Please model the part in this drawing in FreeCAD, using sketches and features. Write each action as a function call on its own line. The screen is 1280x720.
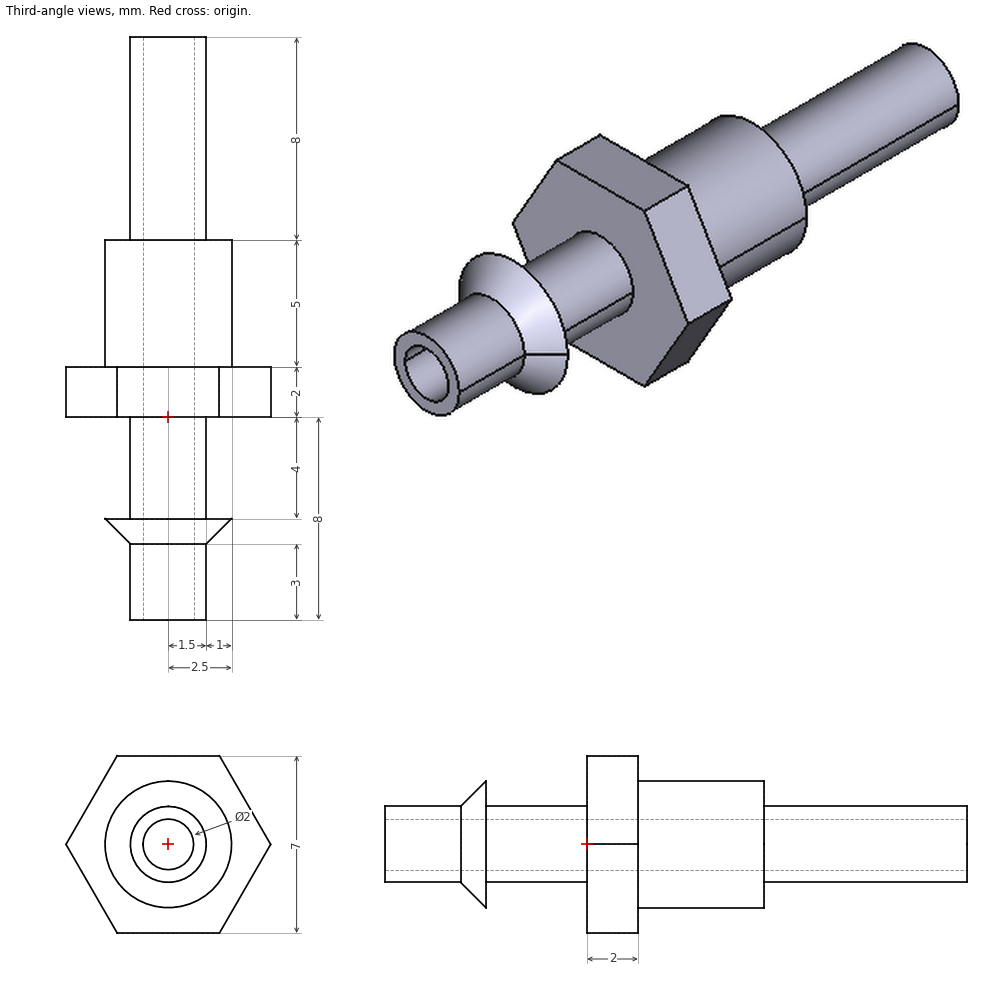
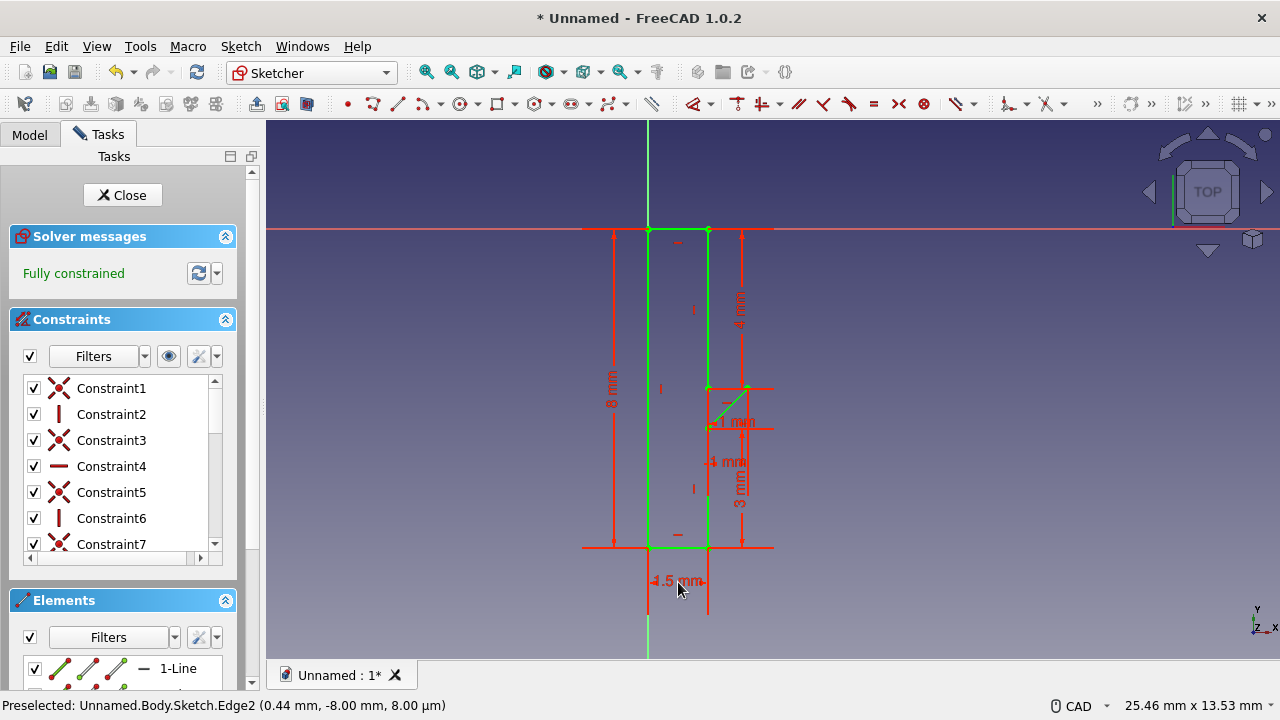
click(123, 195)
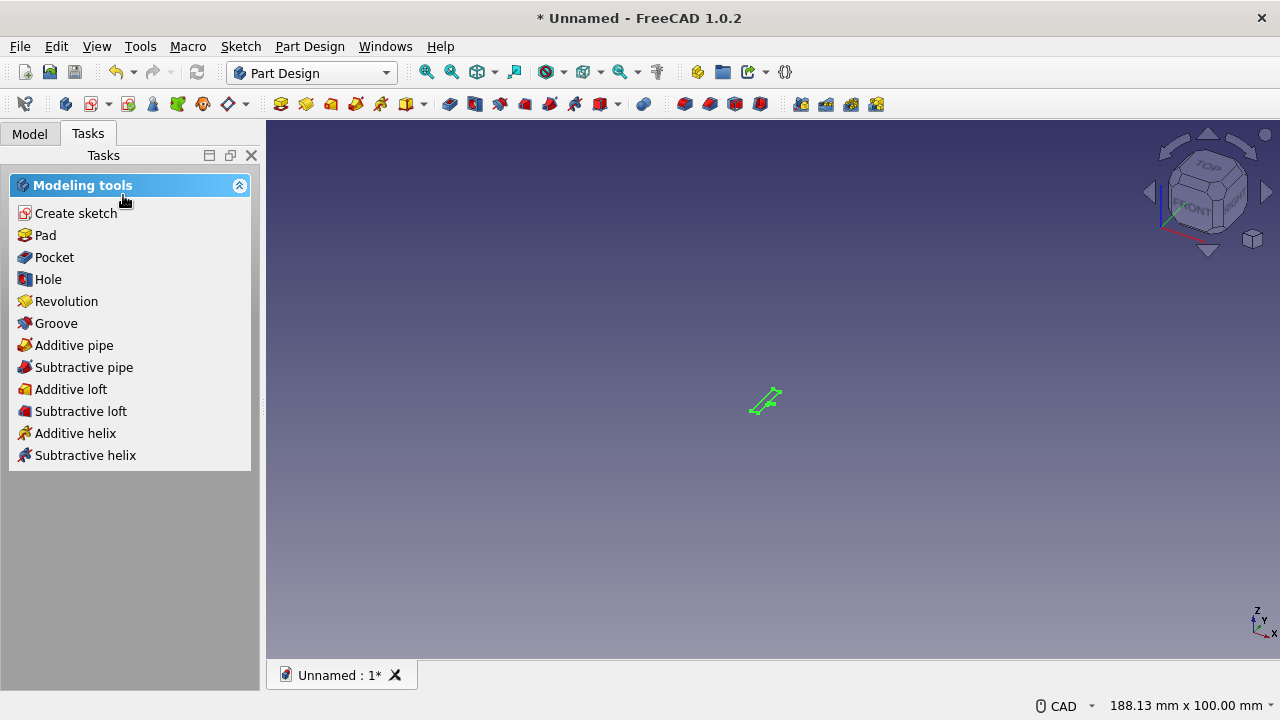
click(306, 104)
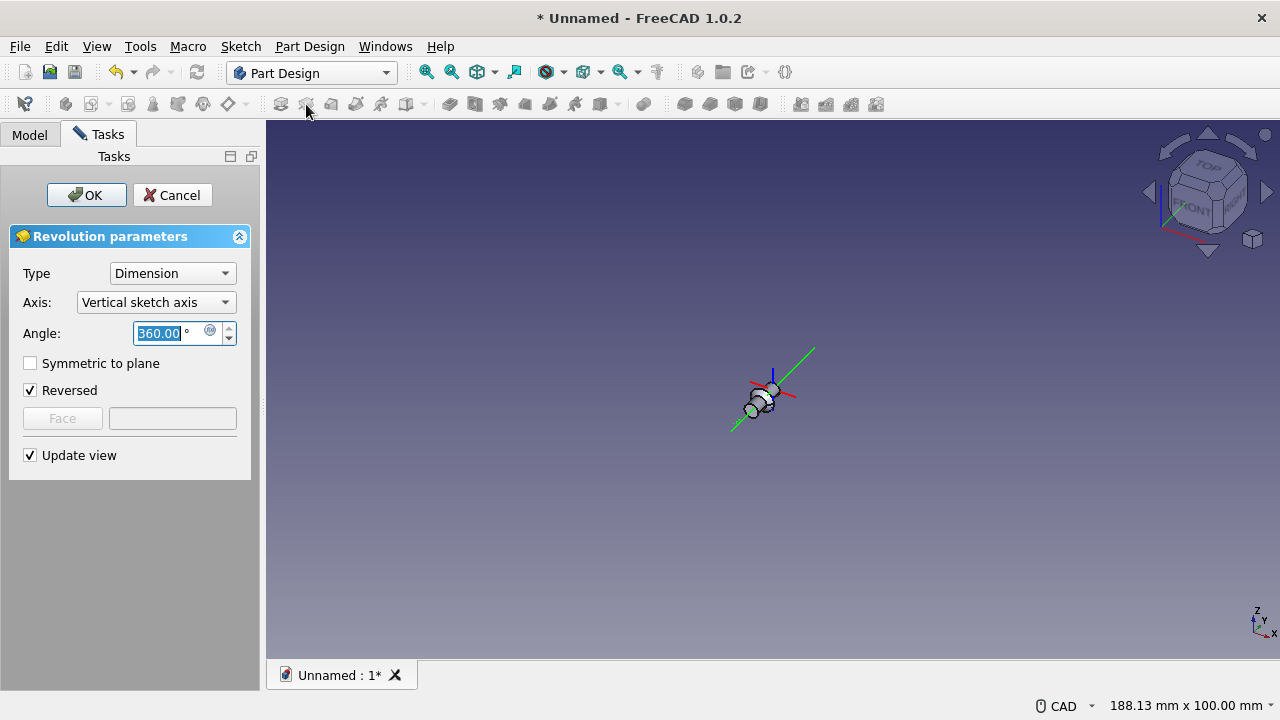
click(87, 195)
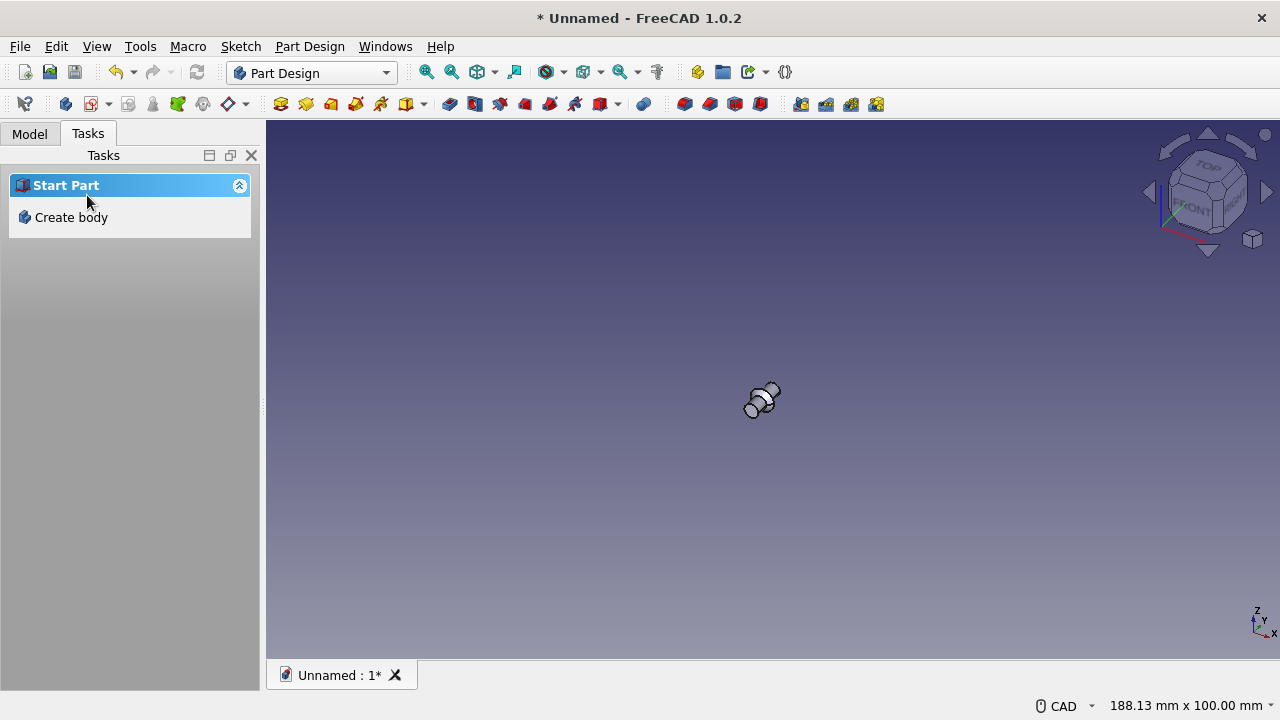
click(427, 72)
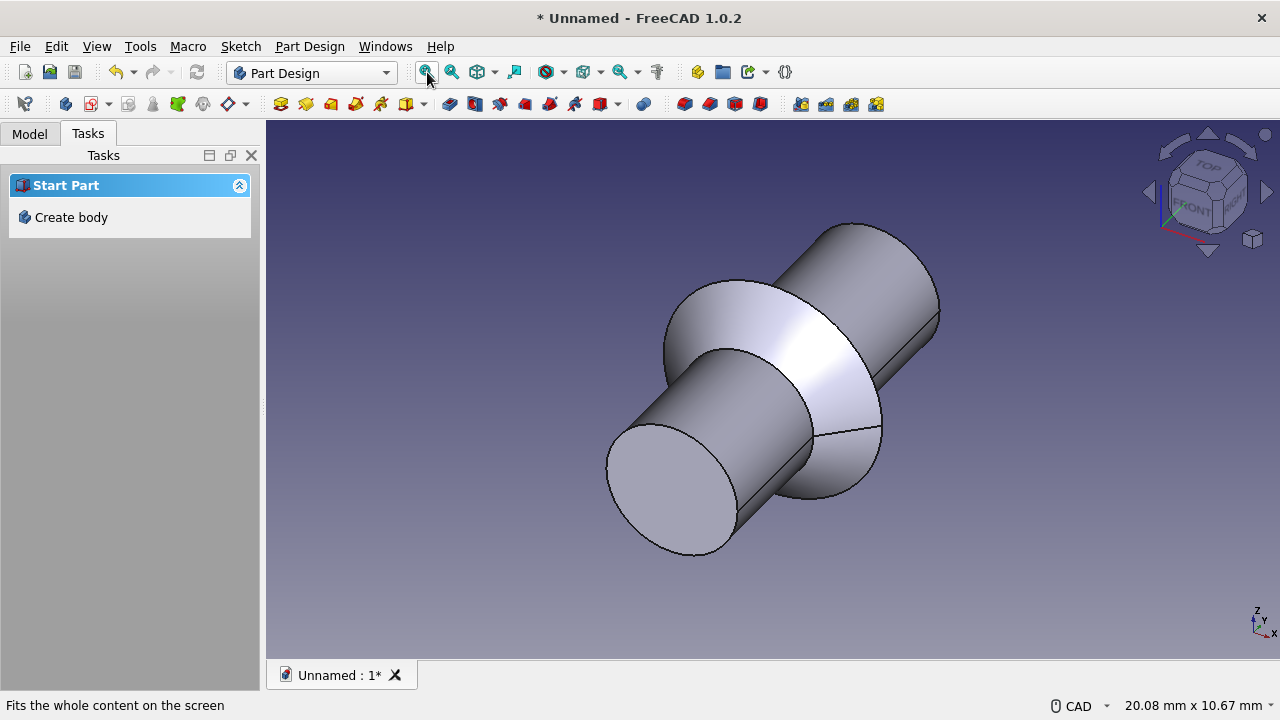
key(4)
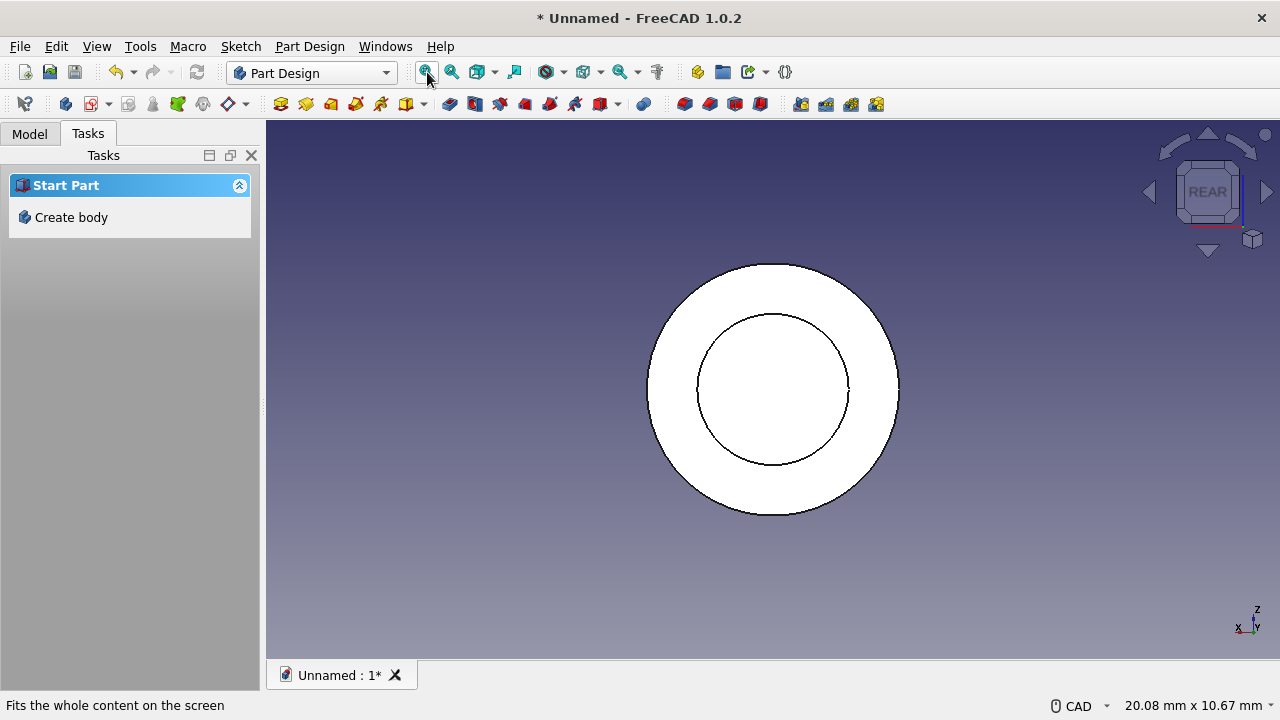
click(773, 388)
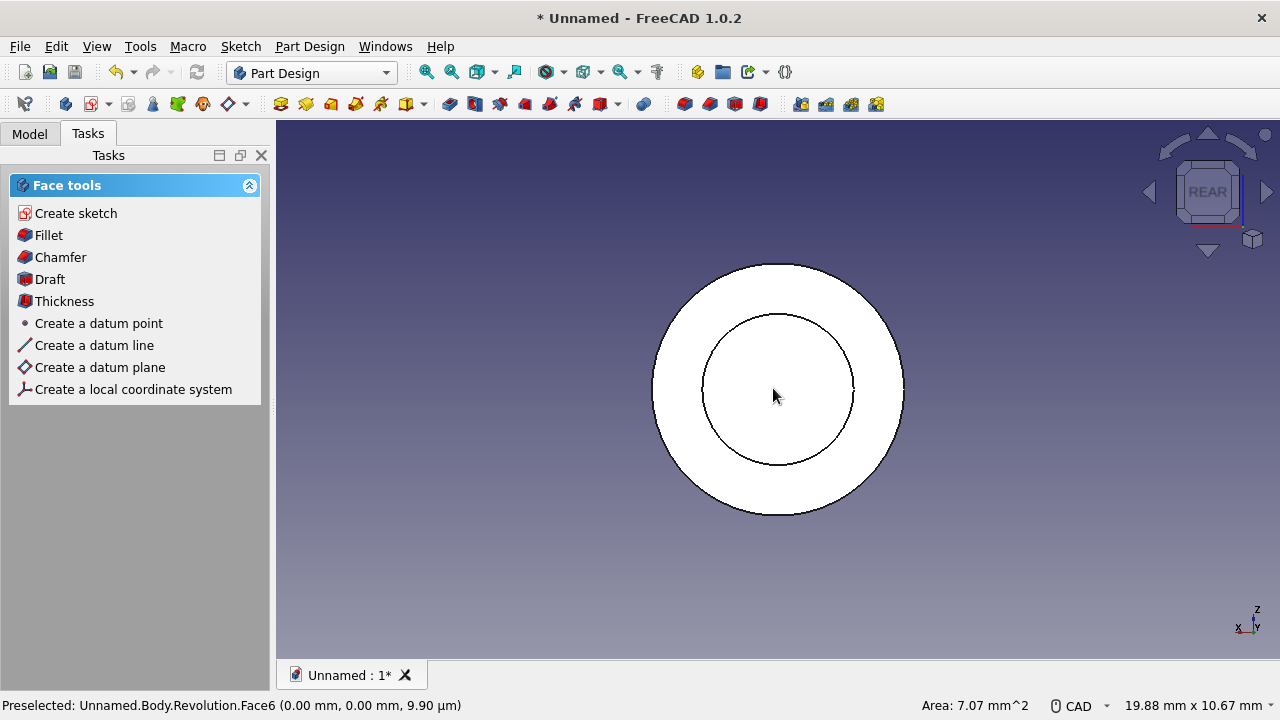
click(90, 104)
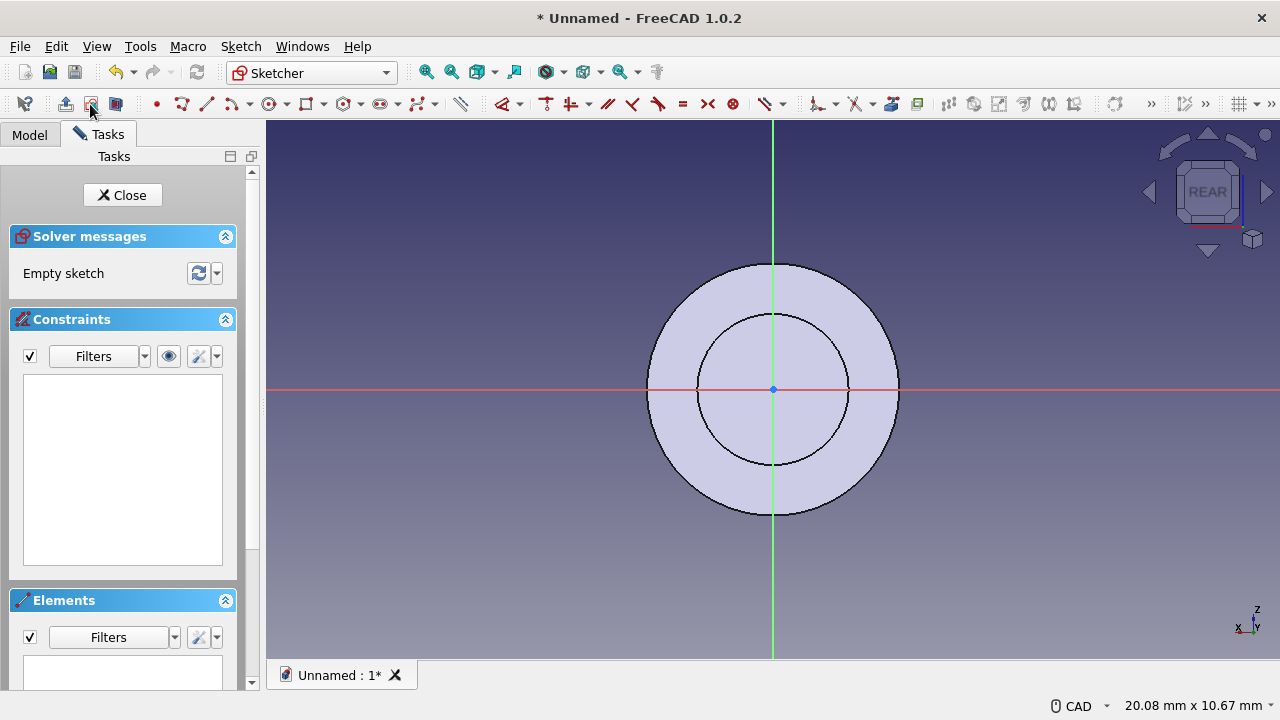
click(342, 104)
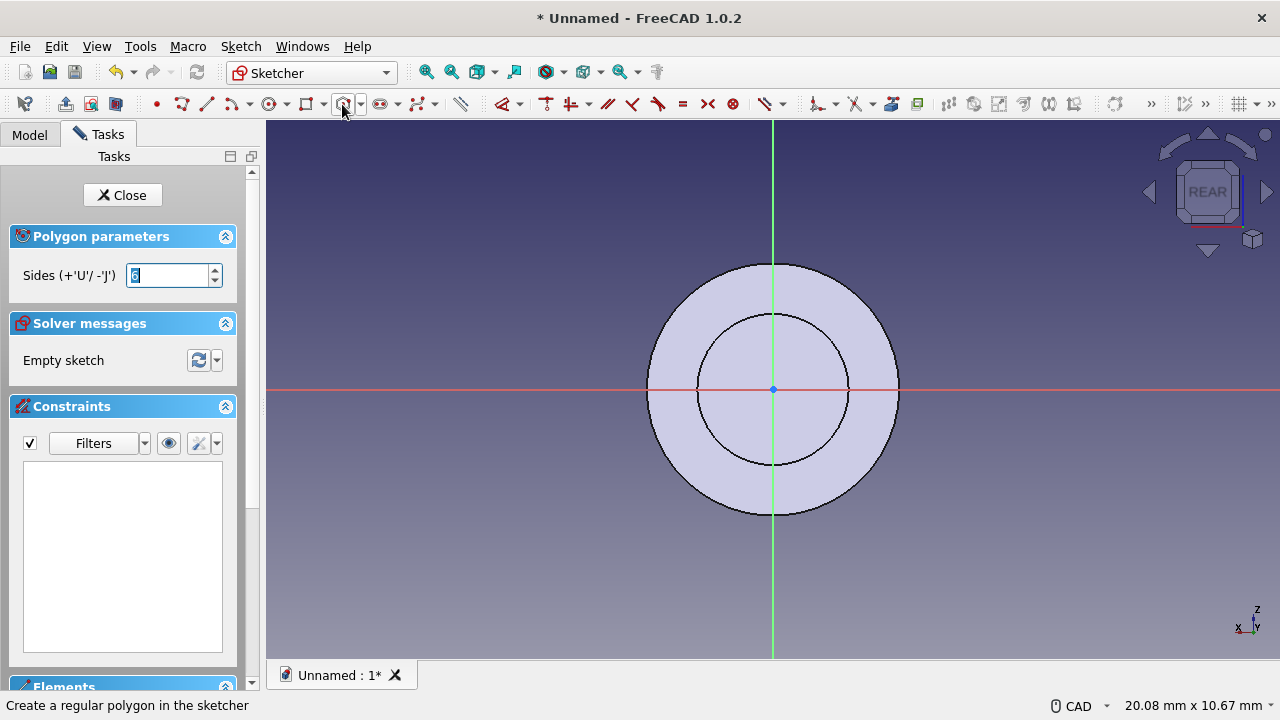
click(773, 389)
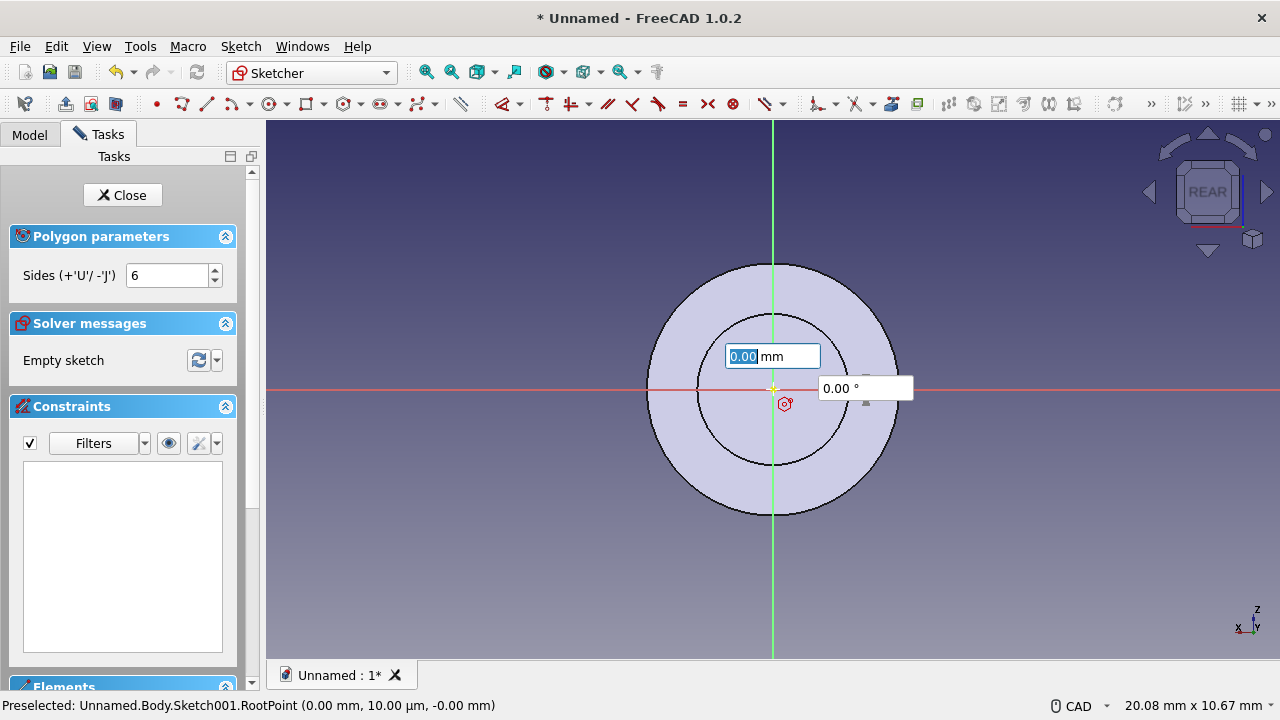
click(569, 389)
key(Escape)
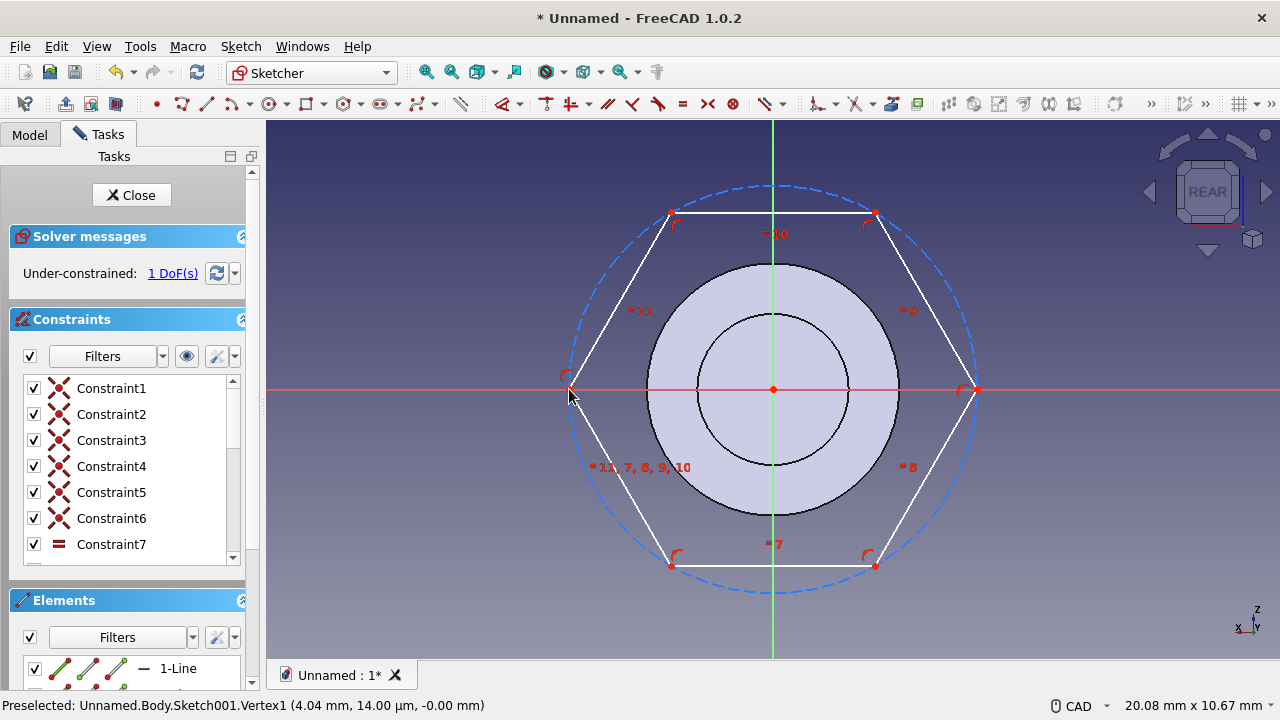
click(502, 104)